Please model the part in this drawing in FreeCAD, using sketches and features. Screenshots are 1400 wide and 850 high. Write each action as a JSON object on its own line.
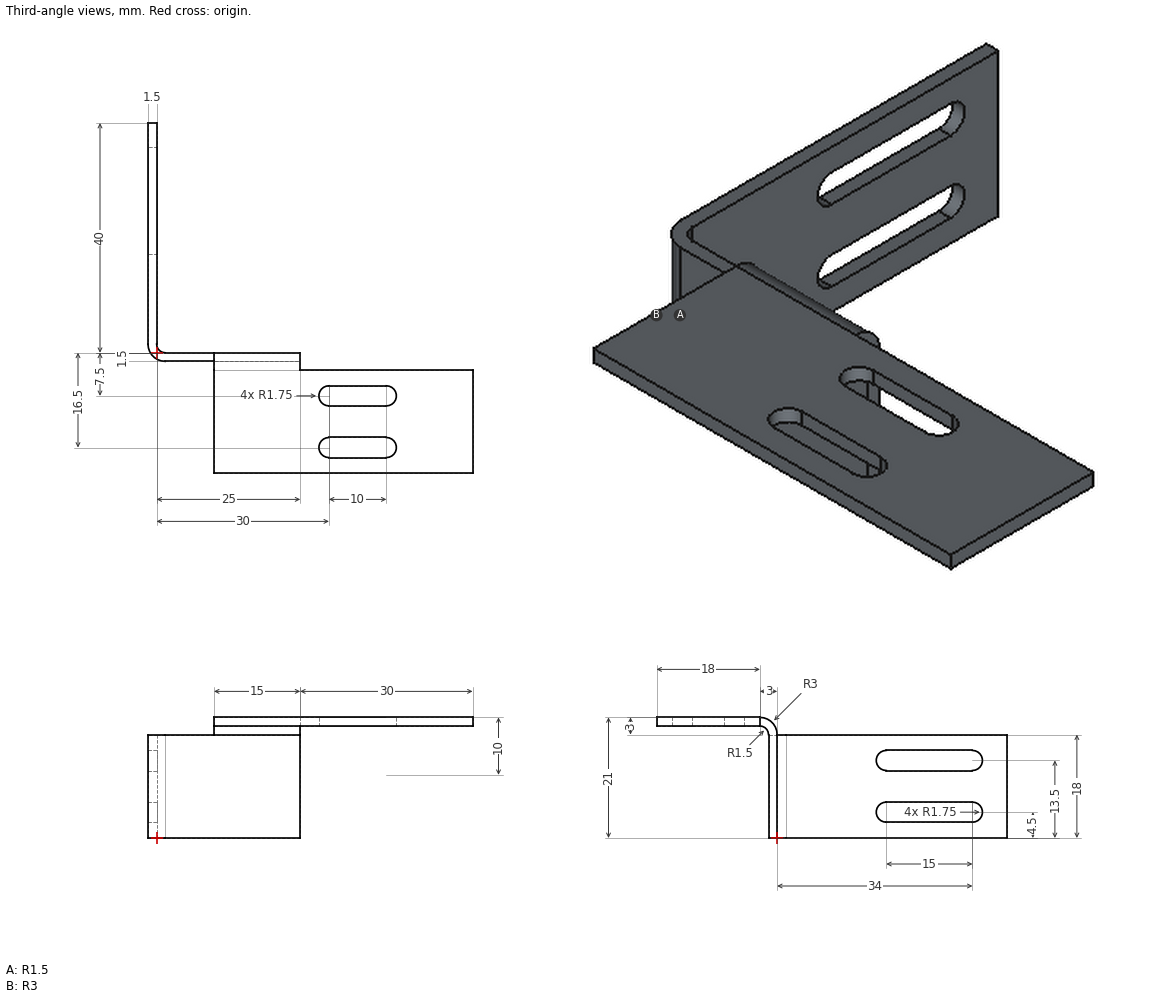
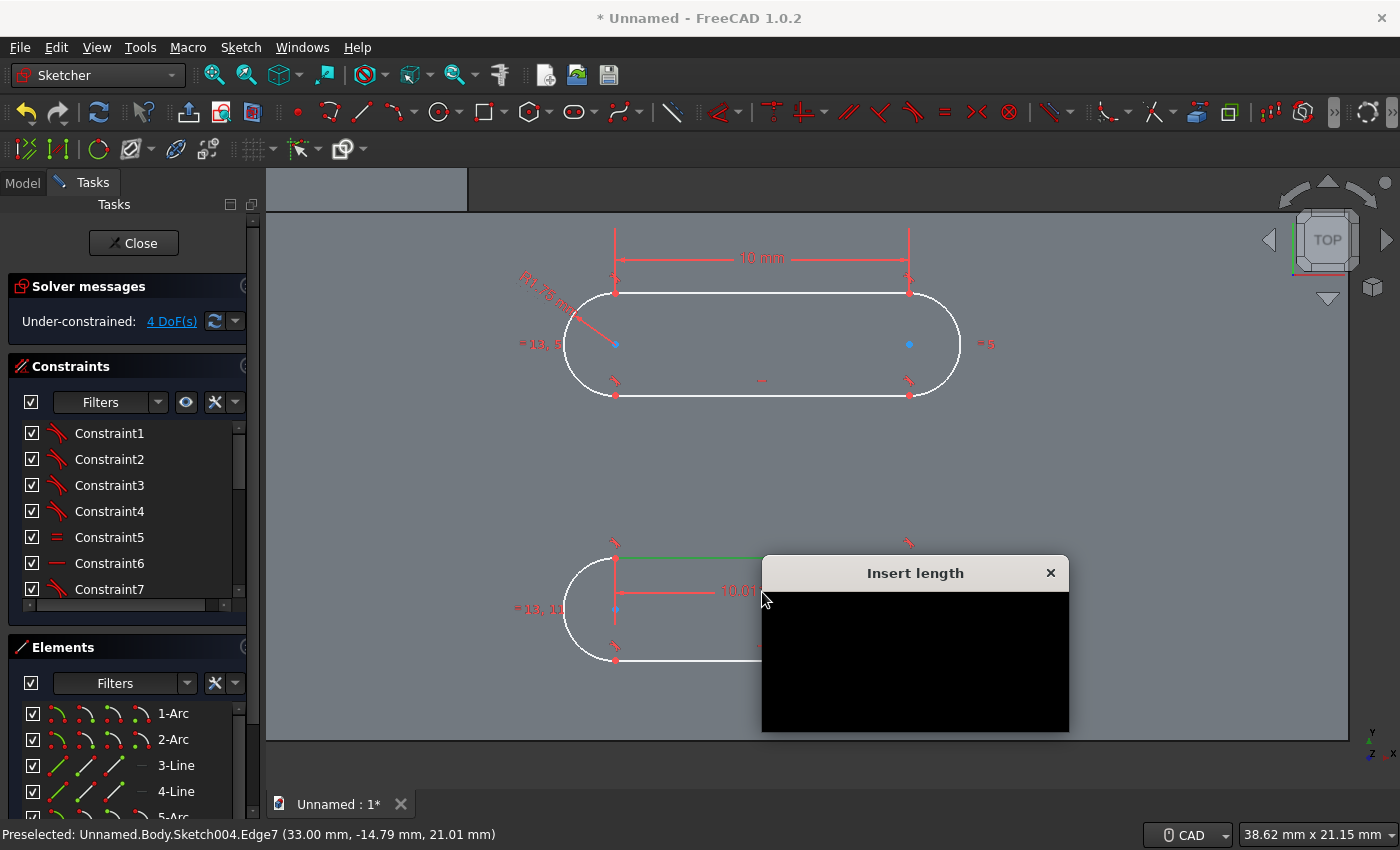
{"action": "type", "text": "10"}
{"action": "key", "text": "Return"}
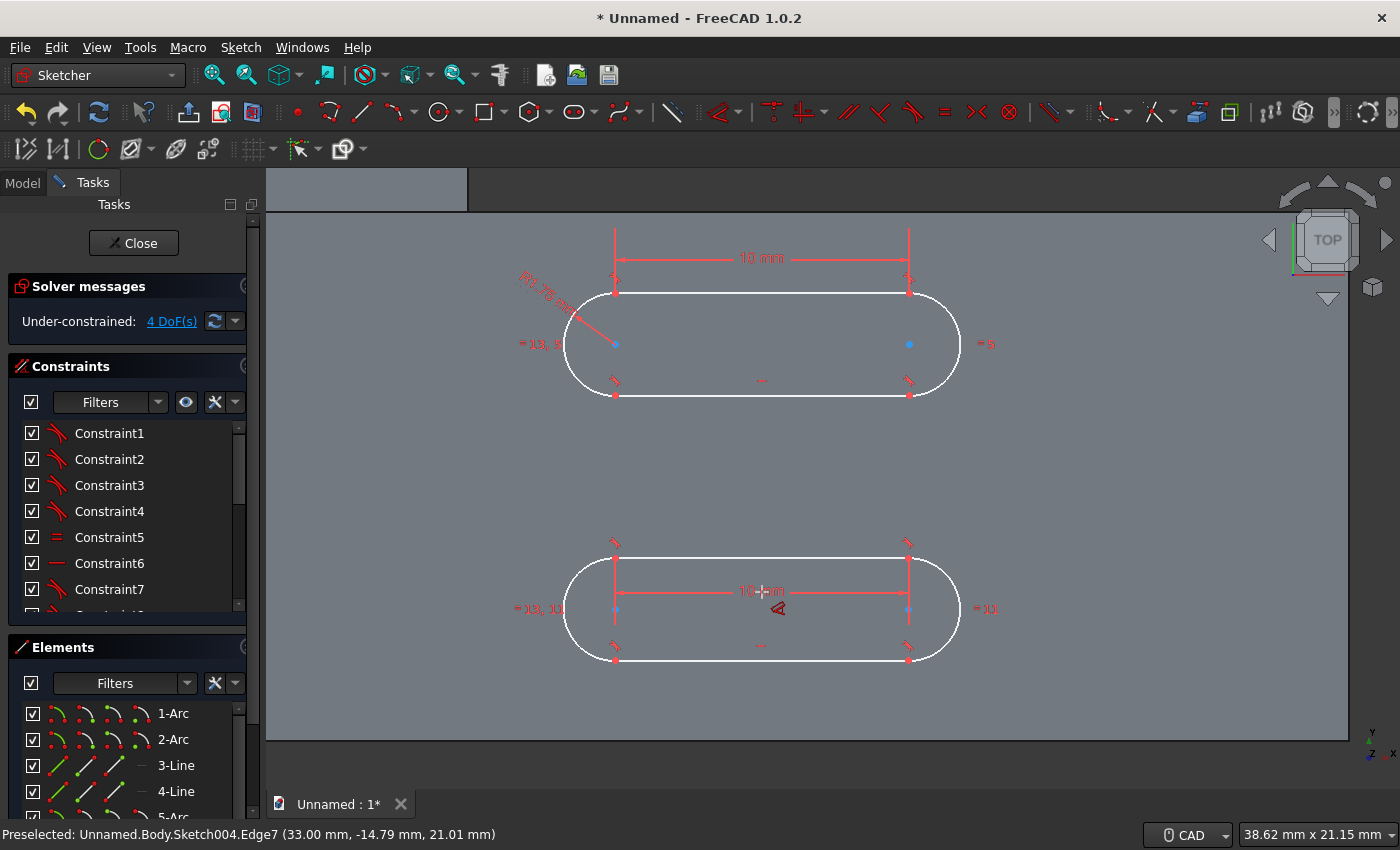
{"action": "left_click", "coordinate": [615, 293]}
{"action": "left_click", "coordinate": [455, 327]}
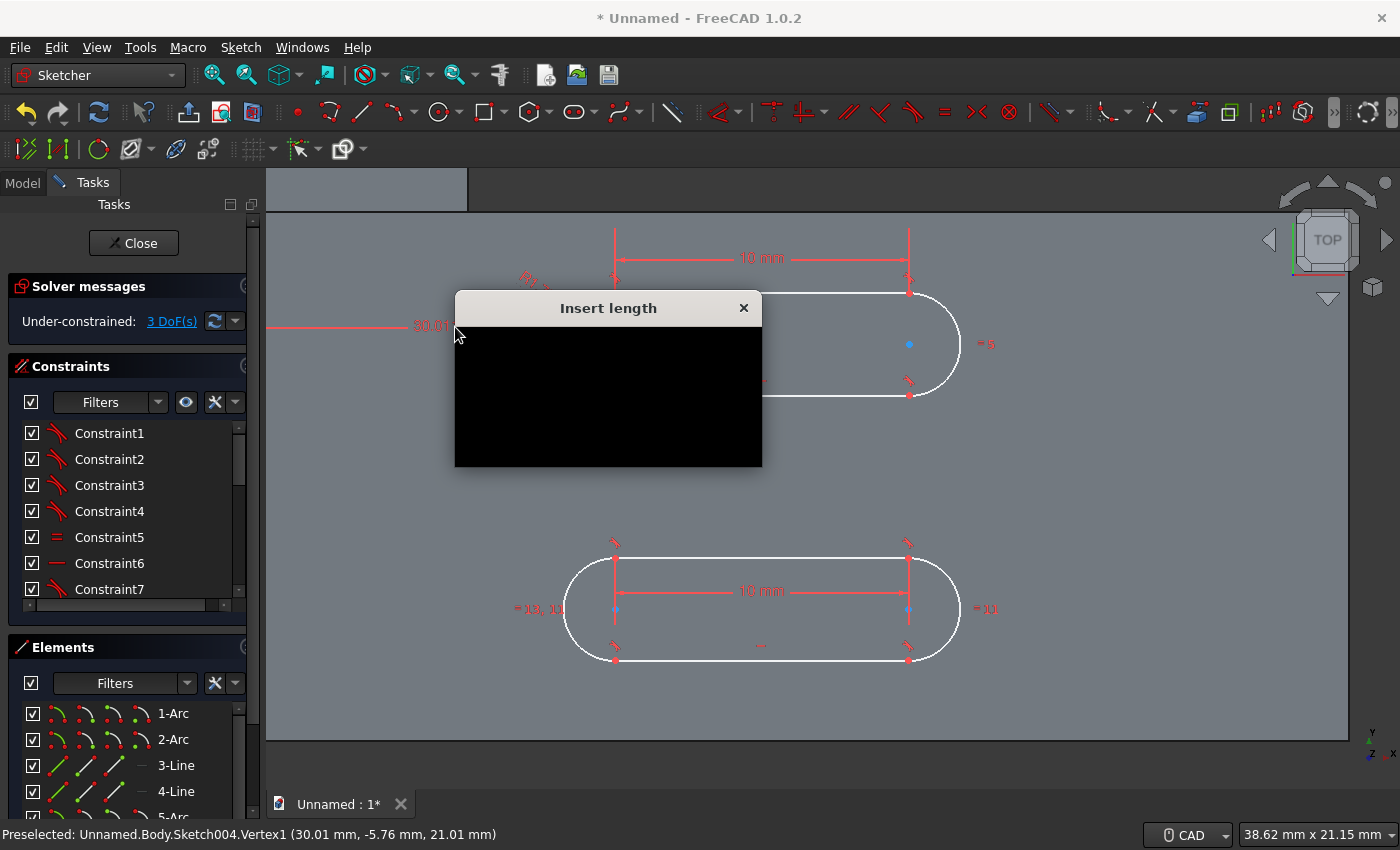
{"action": "type", "text": "30"}
{"action": "key", "text": "Return"}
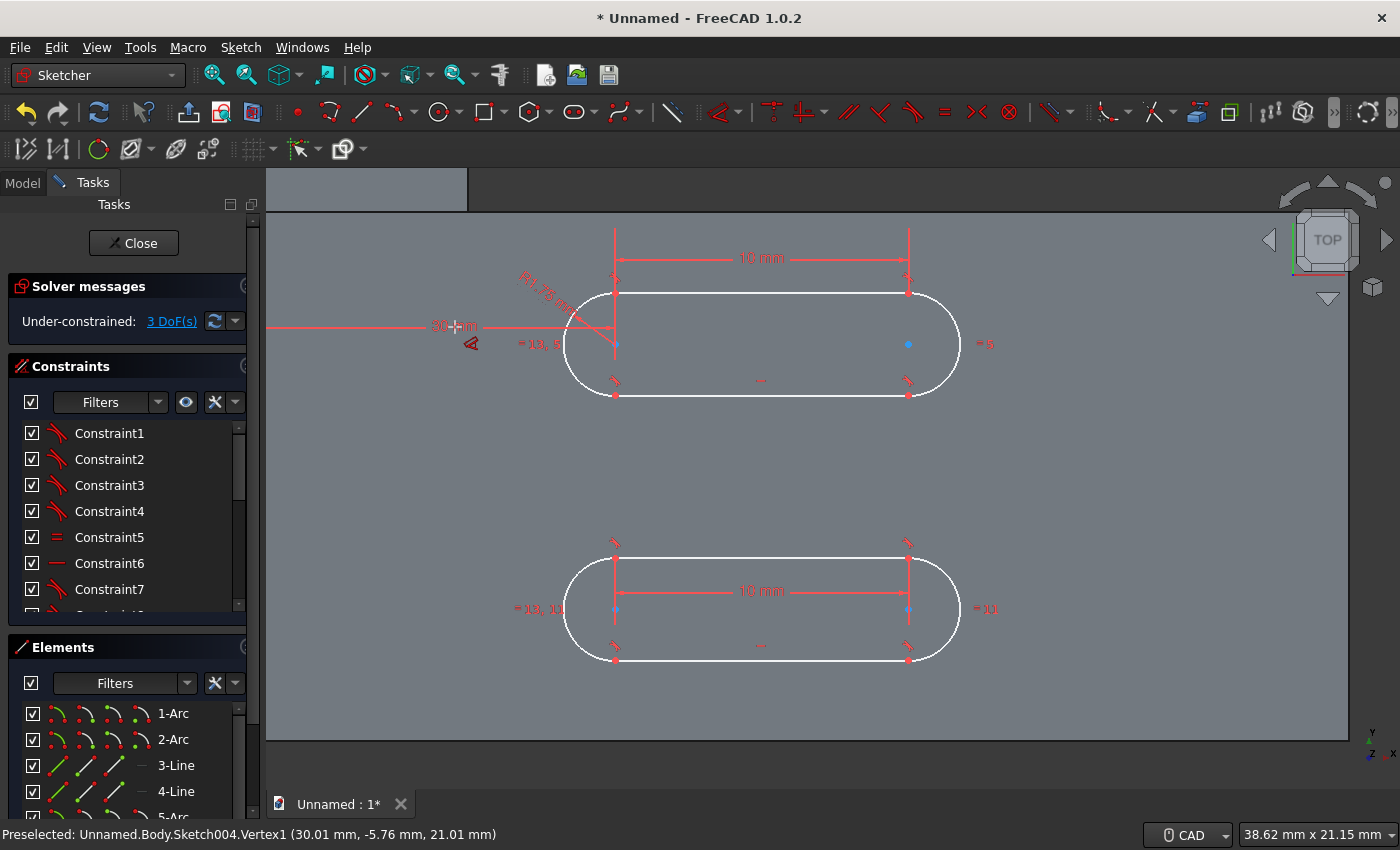
{"action": "left_click", "coordinate": [615, 558]}
{"action": "left_click", "coordinate": [455, 592]}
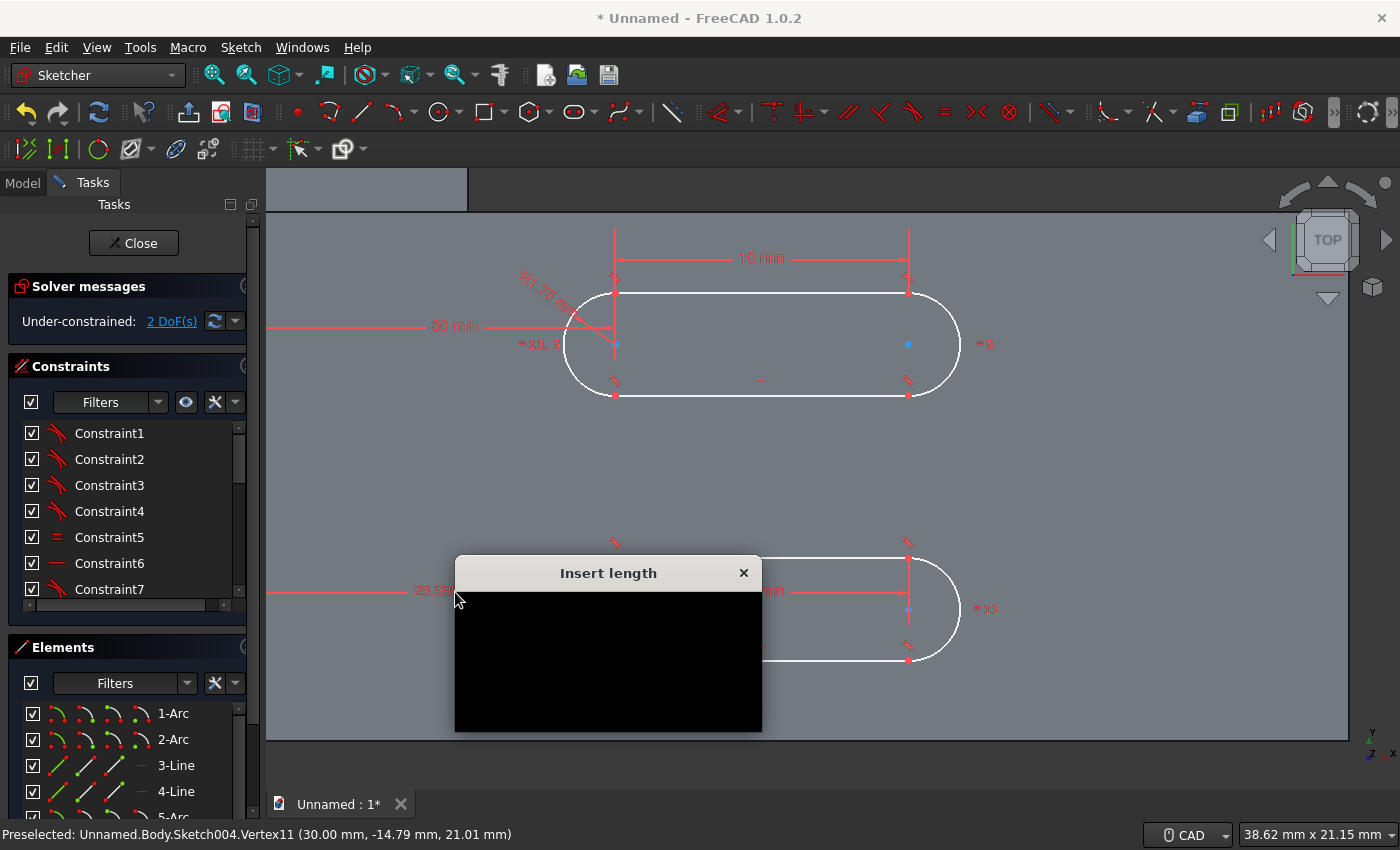
{"action": "type", "text": "30"}
{"action": "key", "text": "Return"}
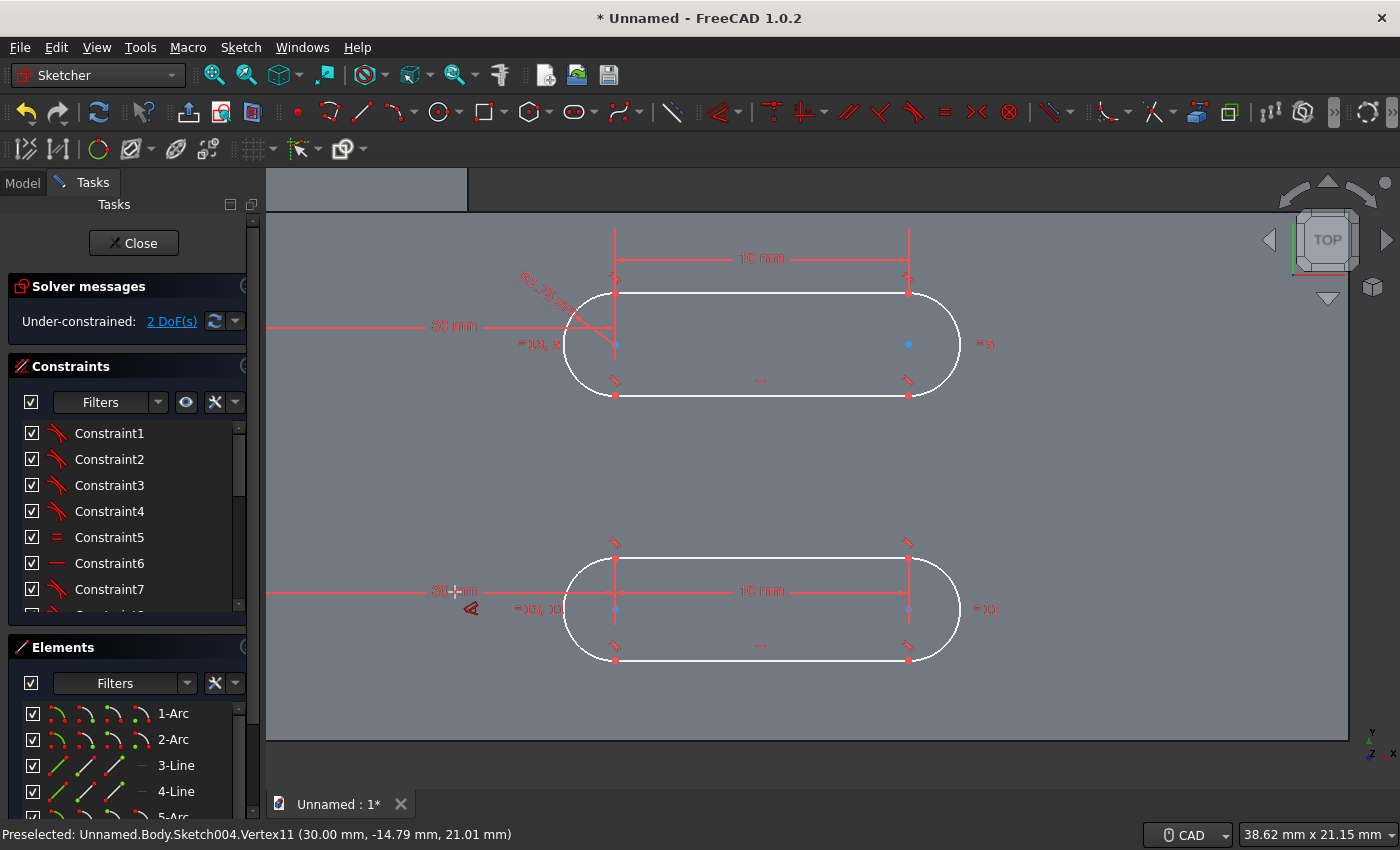
{"action": "left_click", "coordinate": [615, 345]}
{"action": "left_click", "coordinate": [649, 270]}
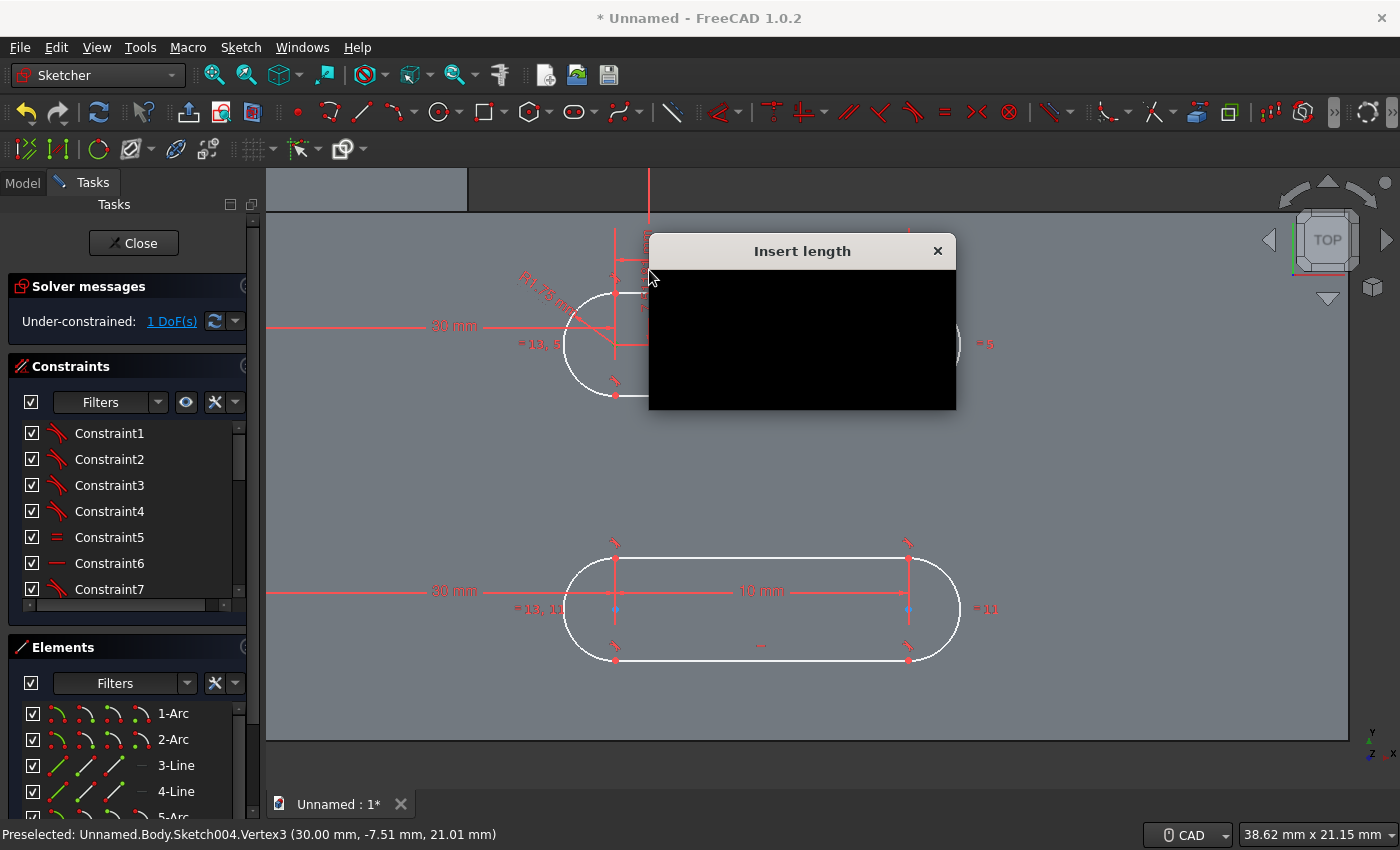
{"action": "type", "text": "7.5"}
{"action": "key", "text": "Return"}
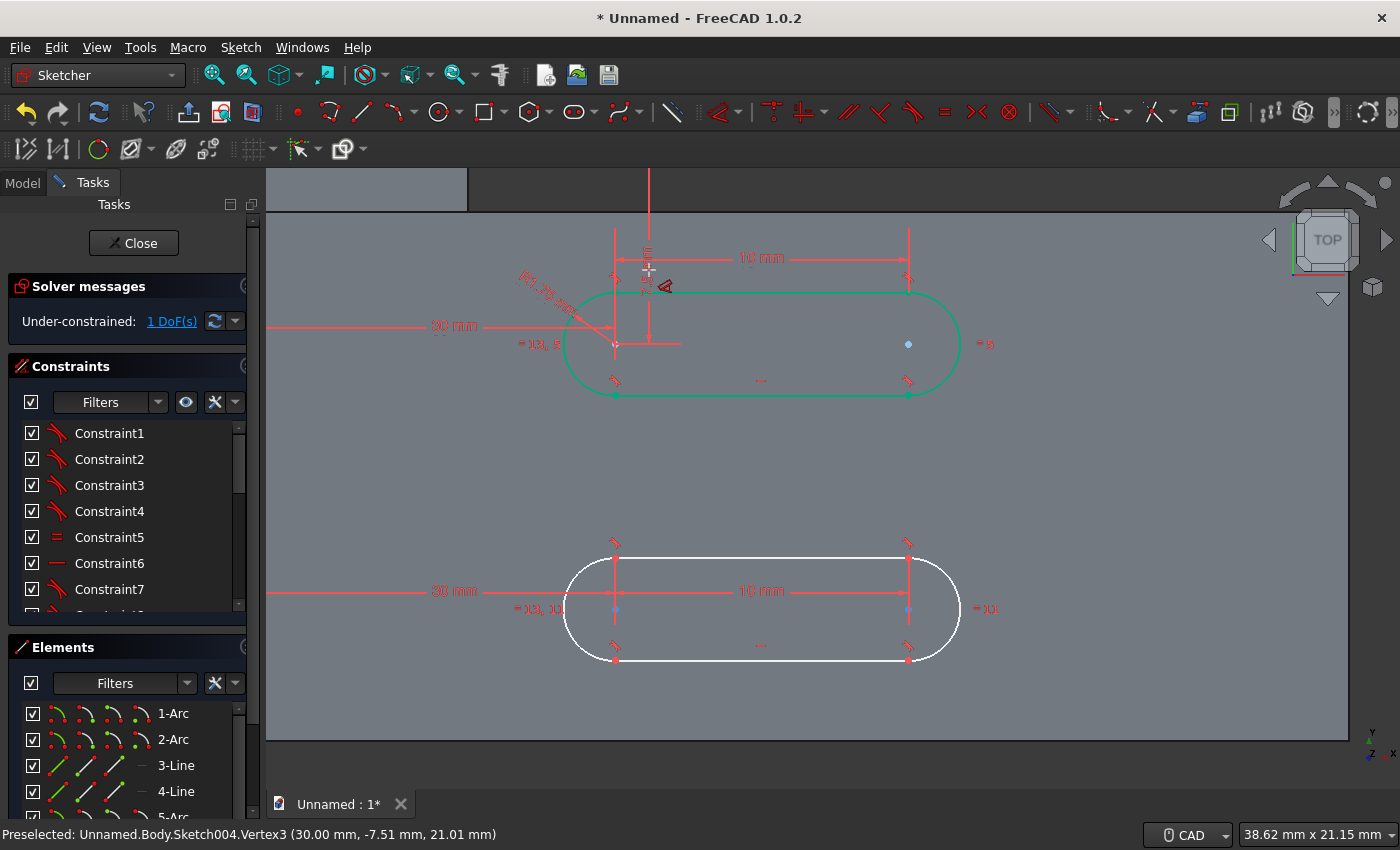
{"action": "left_click", "coordinate": [615, 610]}
{"action": "left_click", "coordinate": [649, 308]}